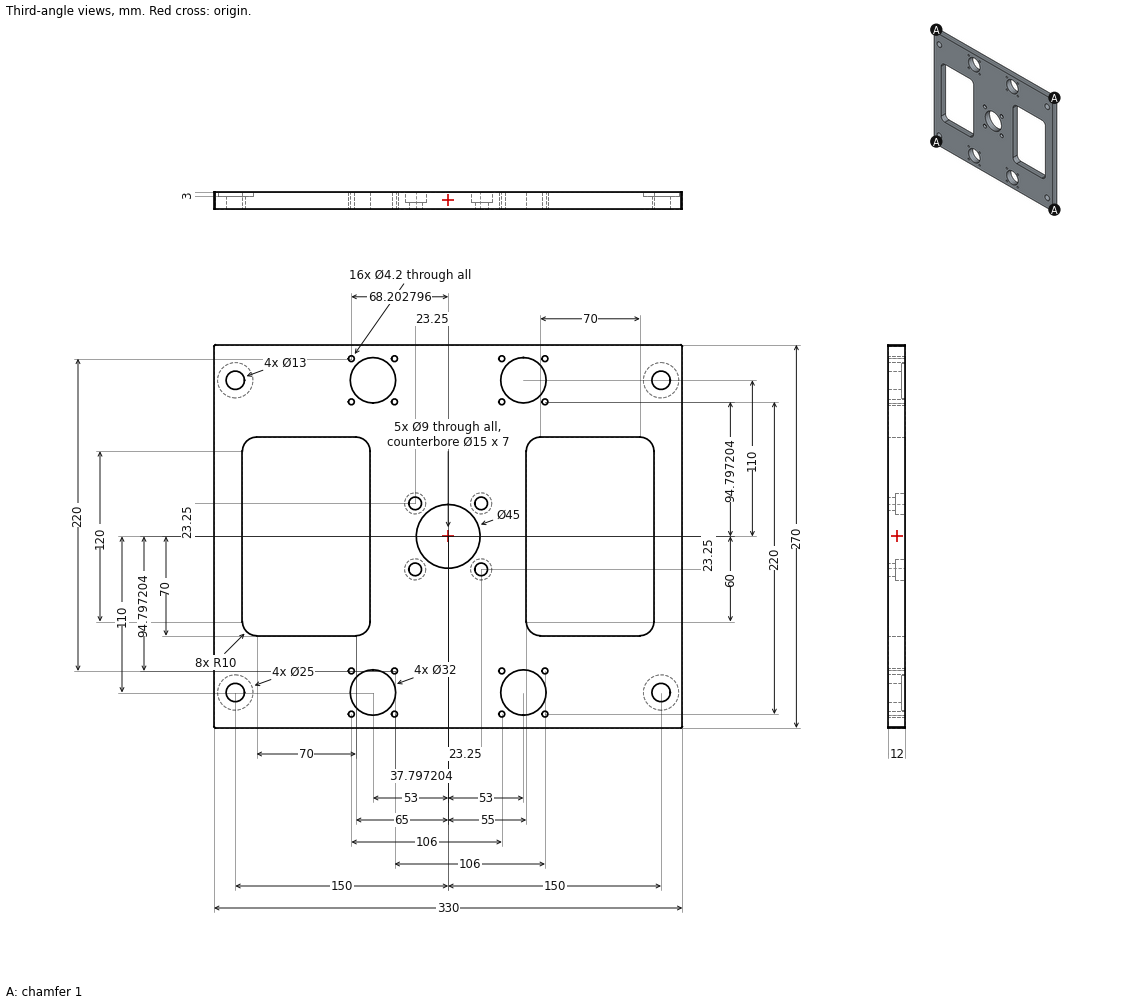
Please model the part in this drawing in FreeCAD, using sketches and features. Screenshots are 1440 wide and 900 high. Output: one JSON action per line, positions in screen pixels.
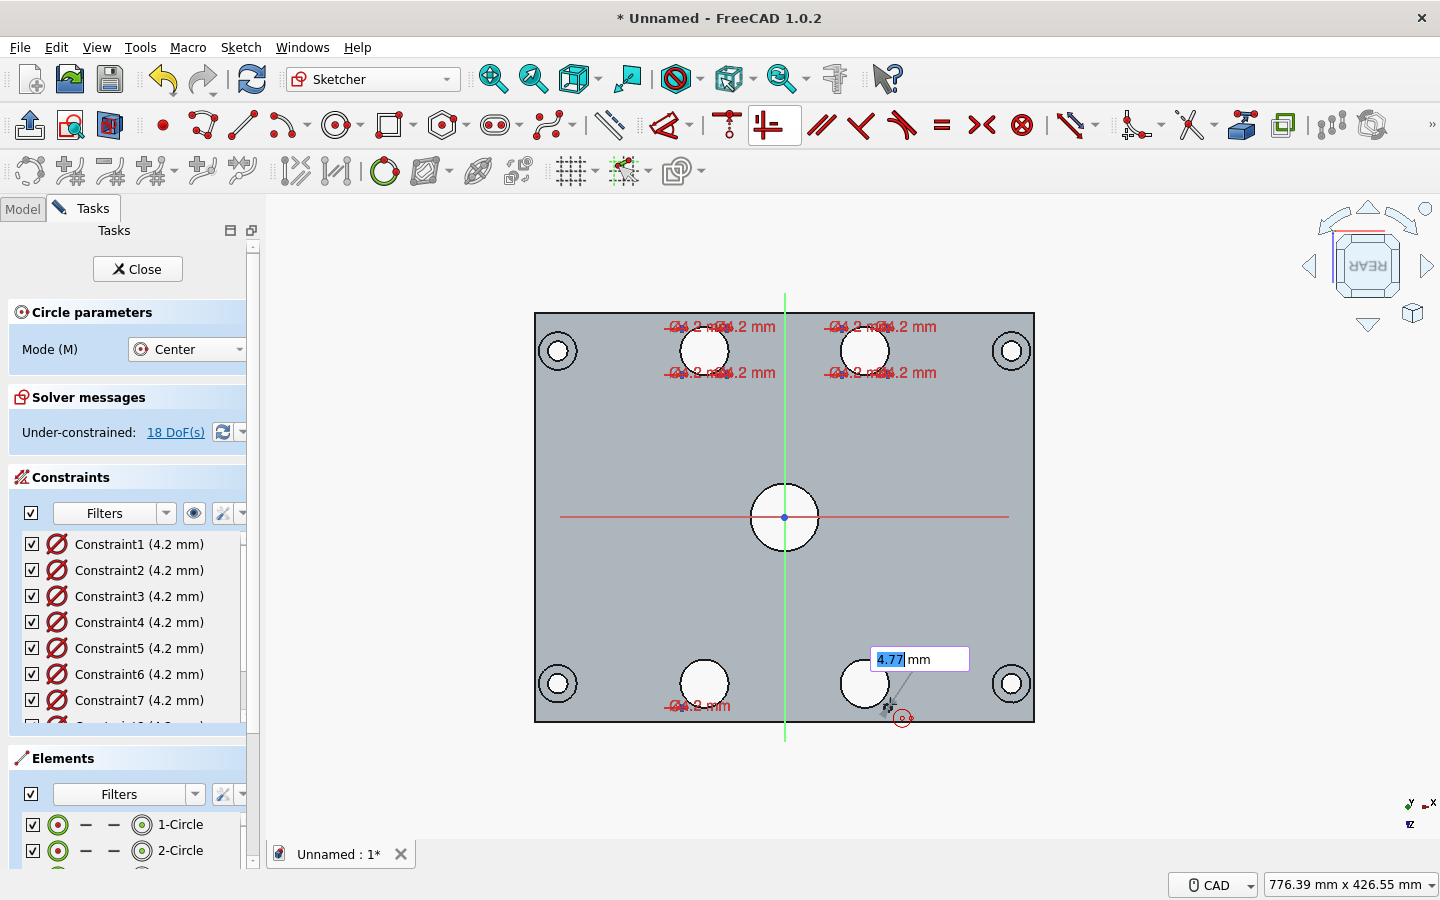
{"action": "type", "text": "4.2"}
{"action": "key", "text": "Return"}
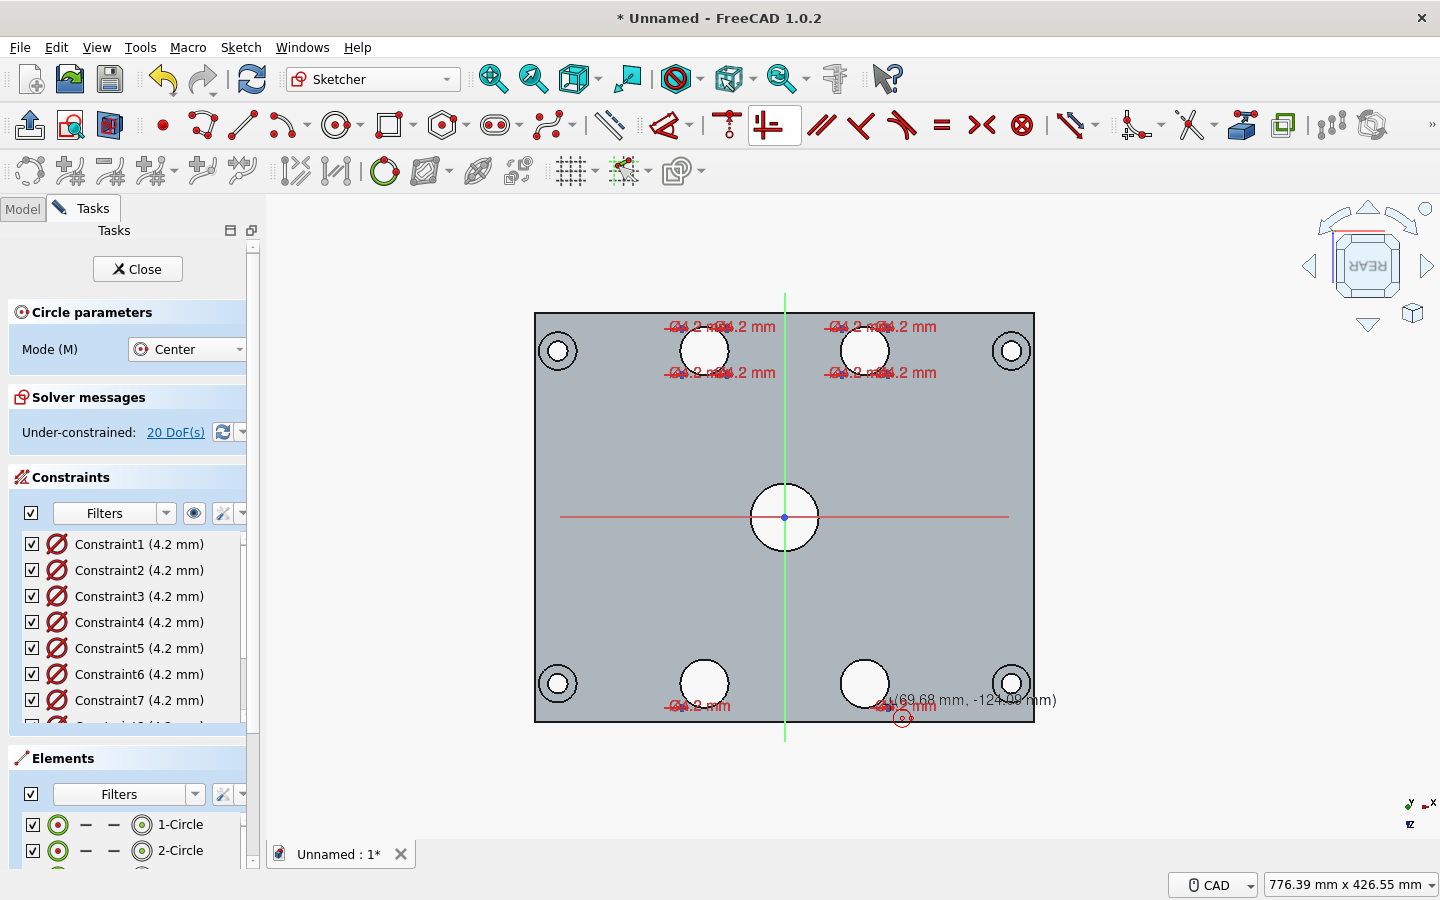
{"action": "scroll", "coordinate": [888, 661], "scroll_direction": "up", "scroll_amount": 10}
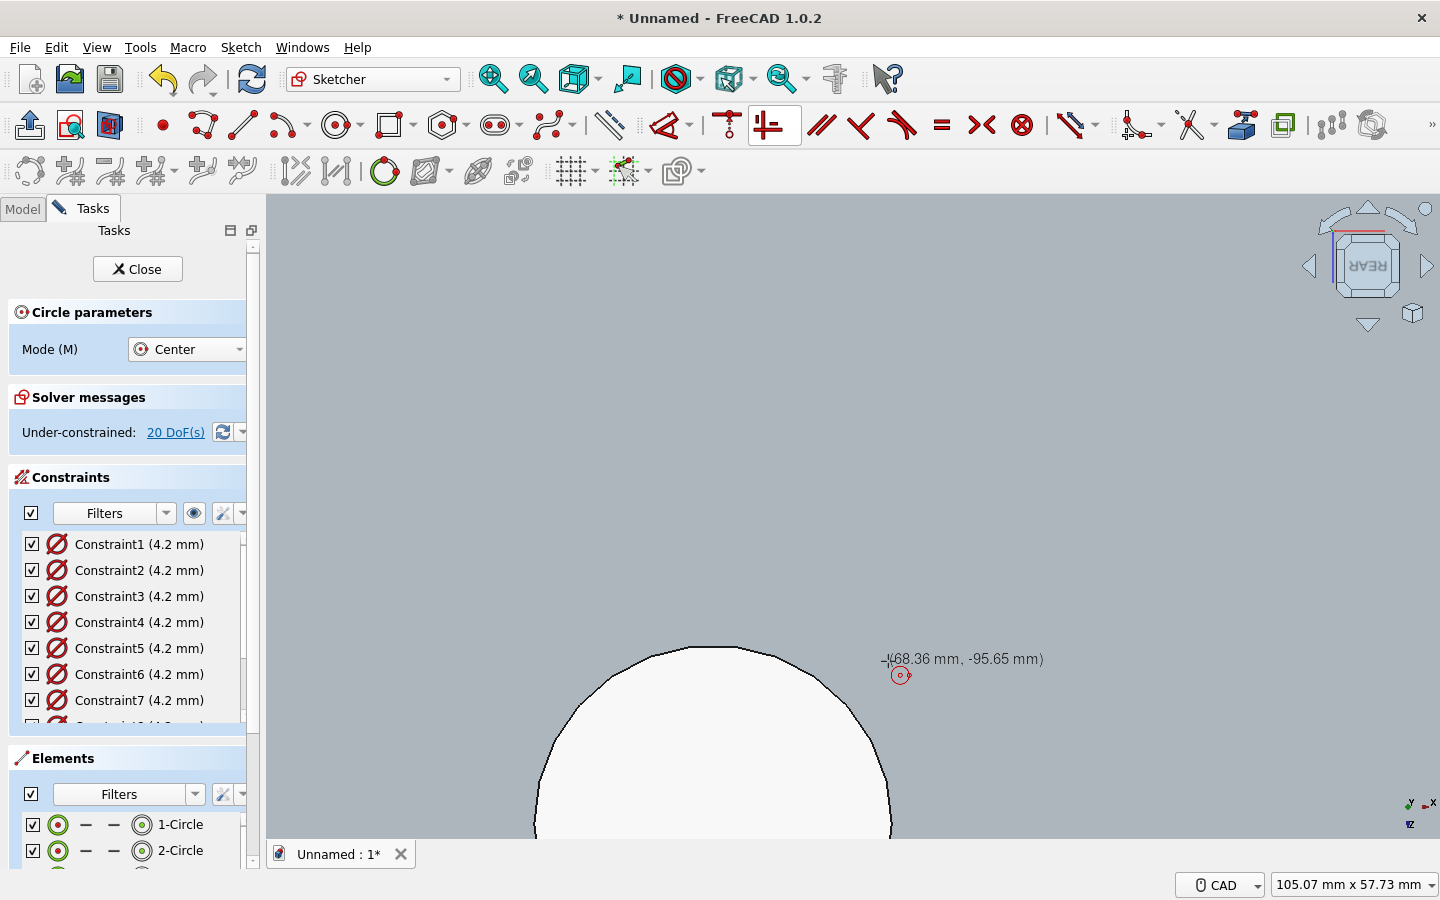
{"action": "scroll", "coordinate": [888, 661], "scroll_direction": "down", "scroll_amount": 10}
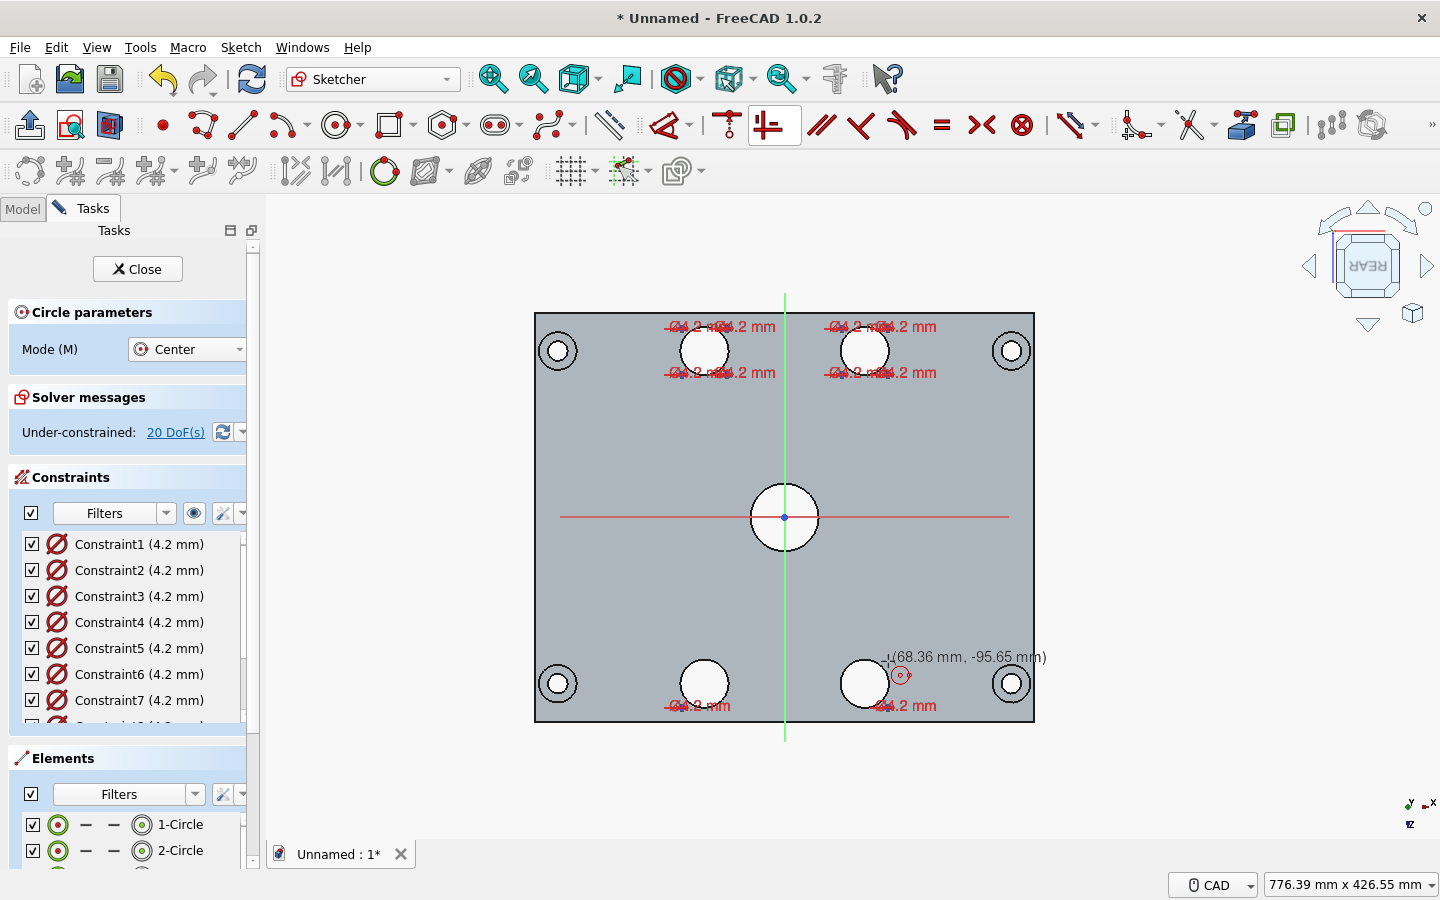
{"action": "left_click", "coordinate": [888, 661]}
{"action": "mouse_move", "coordinate": [890, 658]}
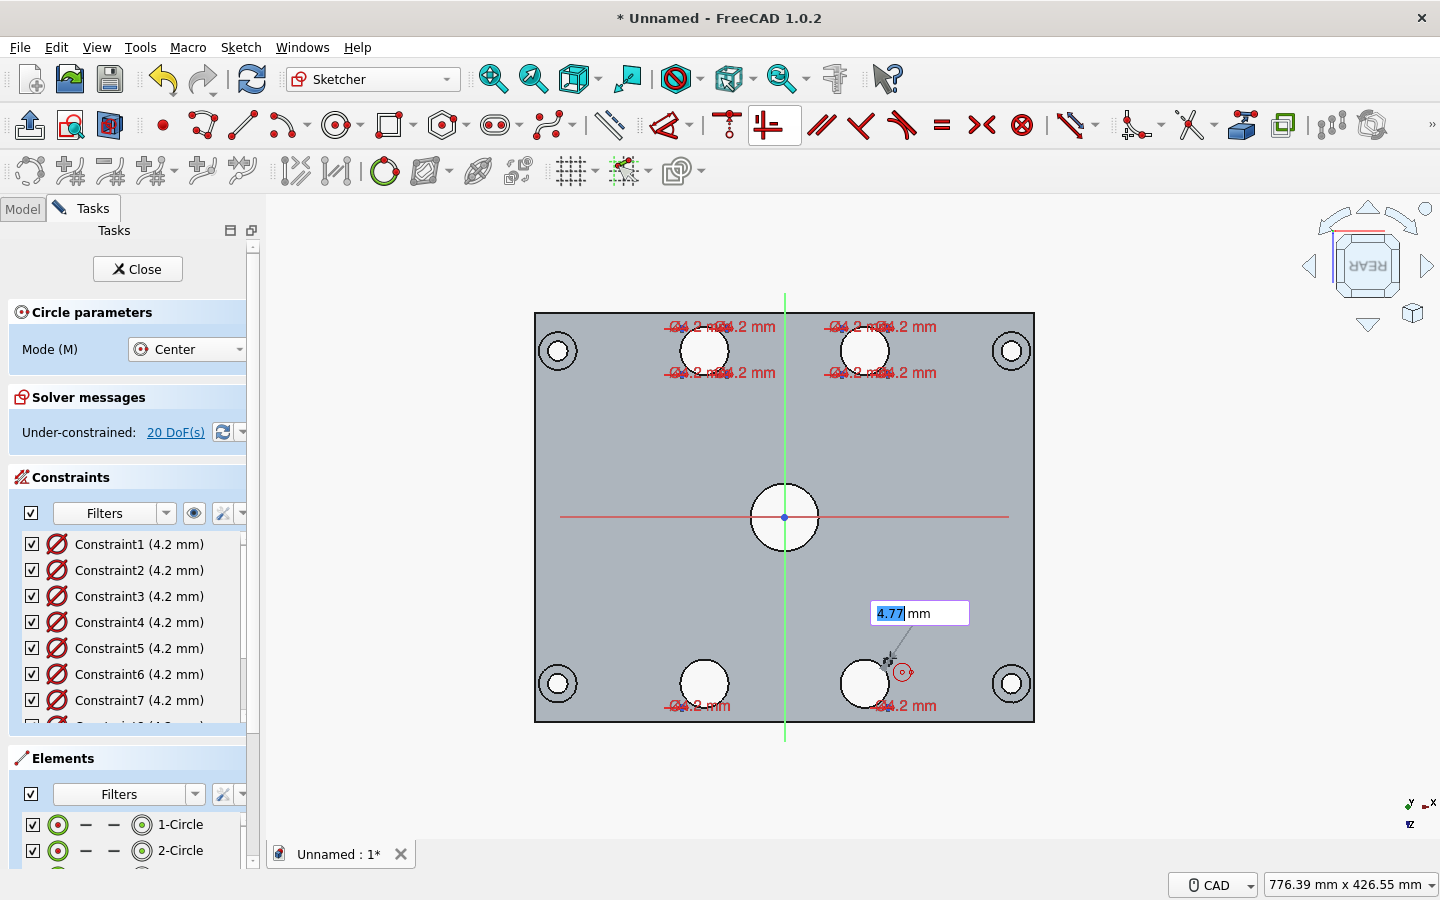
{"action": "type", "text": "4.2"}
{"action": "key", "text": "Return"}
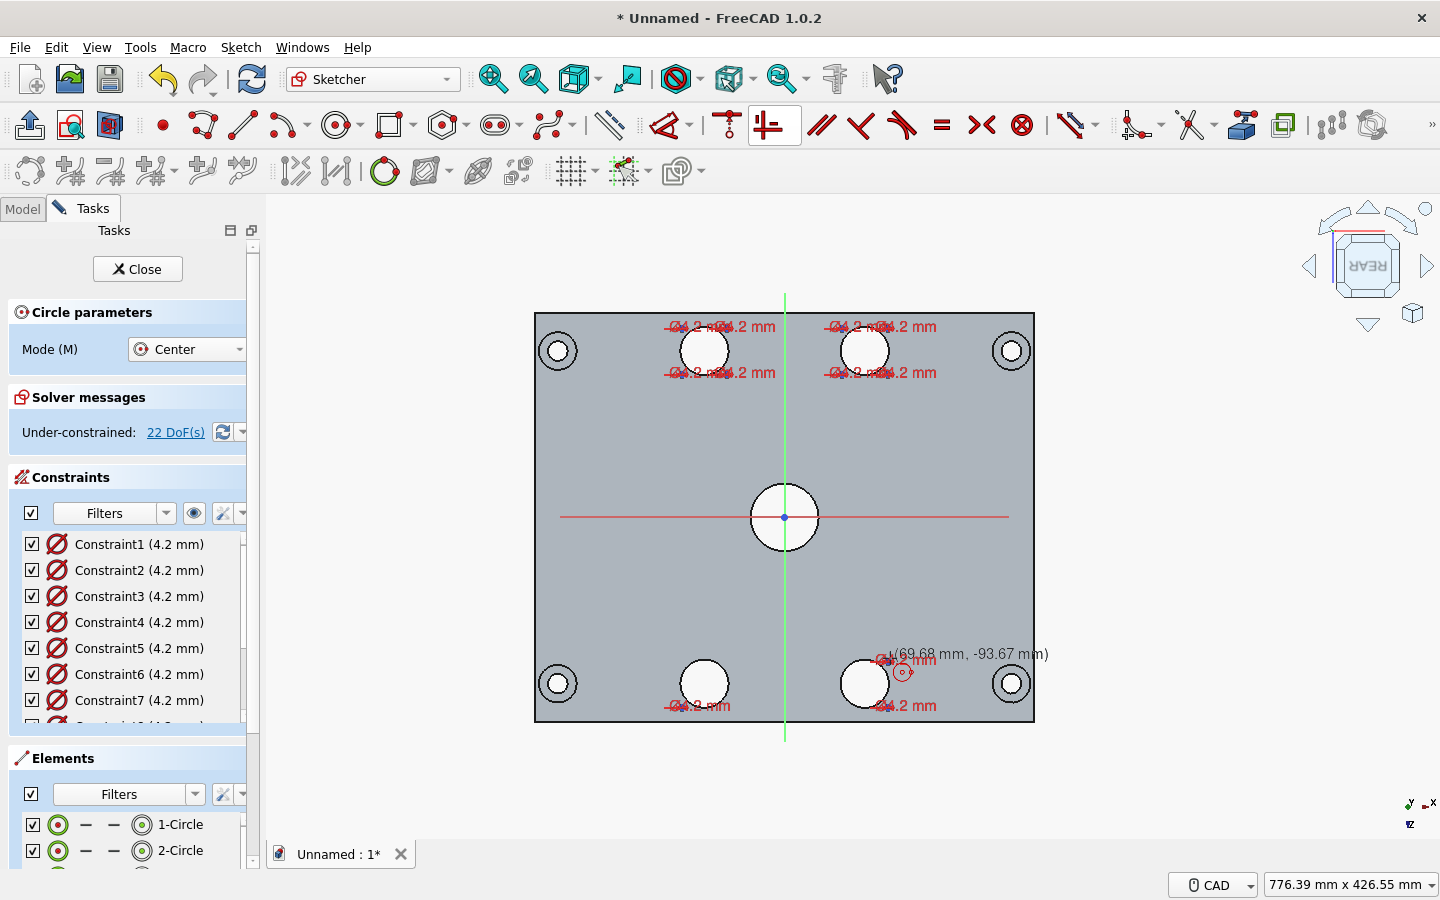
{"action": "scroll", "coordinate": [842, 661], "scroll_direction": "up", "scroll_amount": 10}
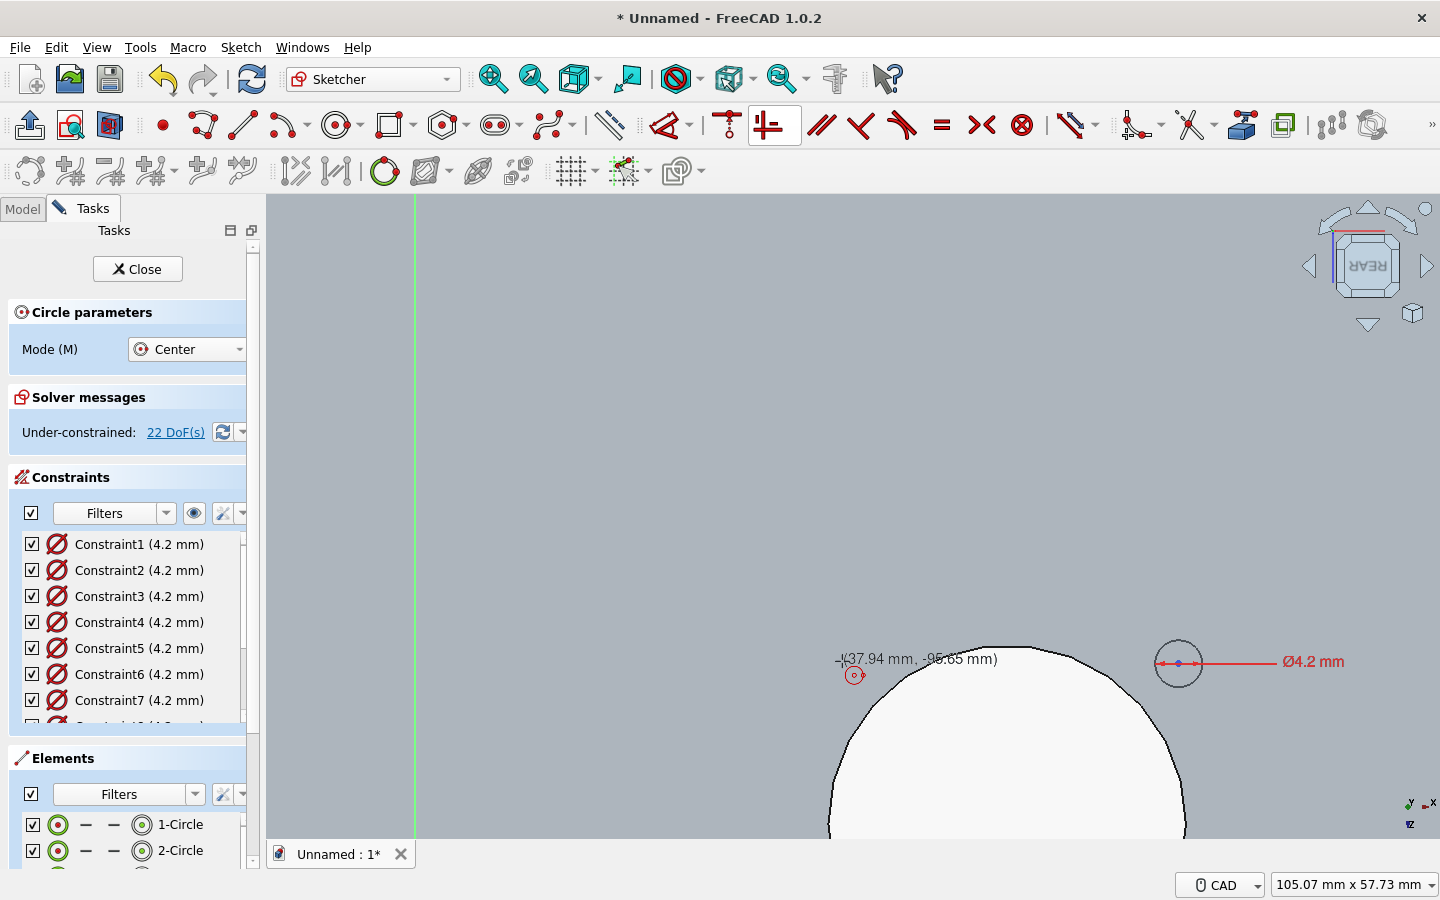
{"action": "scroll", "coordinate": [842, 661], "scroll_direction": "down", "scroll_amount": 10}